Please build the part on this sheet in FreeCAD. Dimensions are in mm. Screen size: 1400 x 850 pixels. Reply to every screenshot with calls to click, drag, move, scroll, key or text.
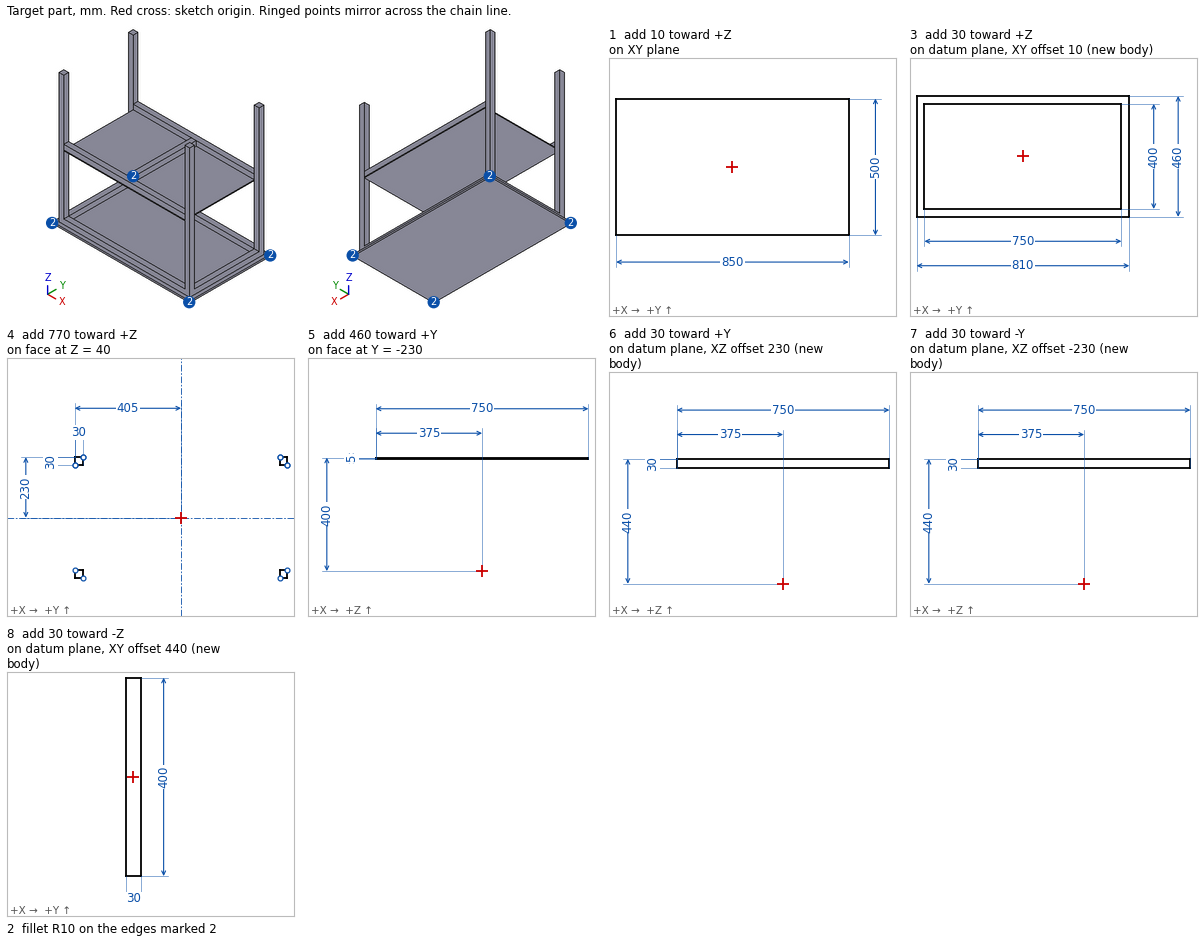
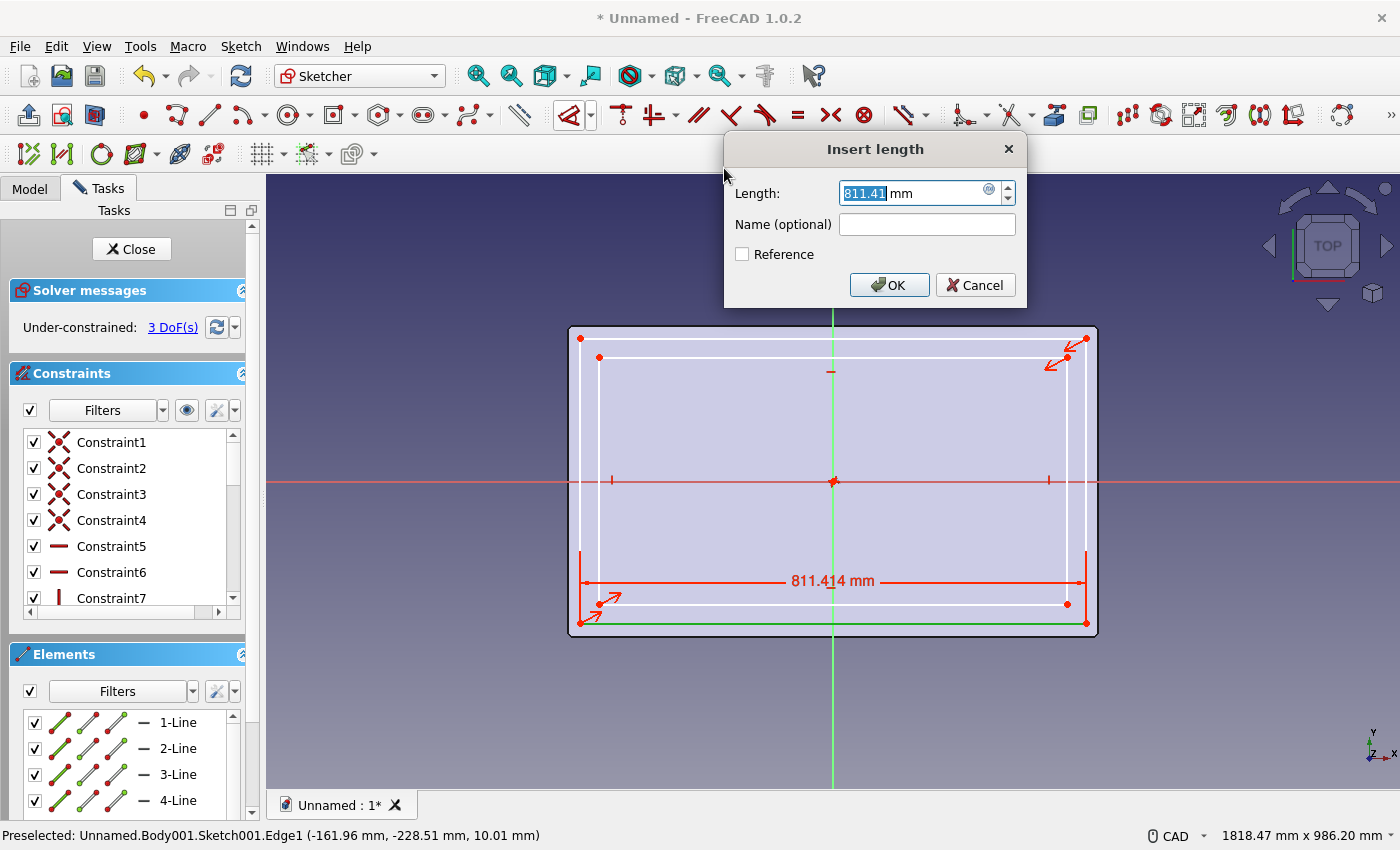
text(810)
key(Return)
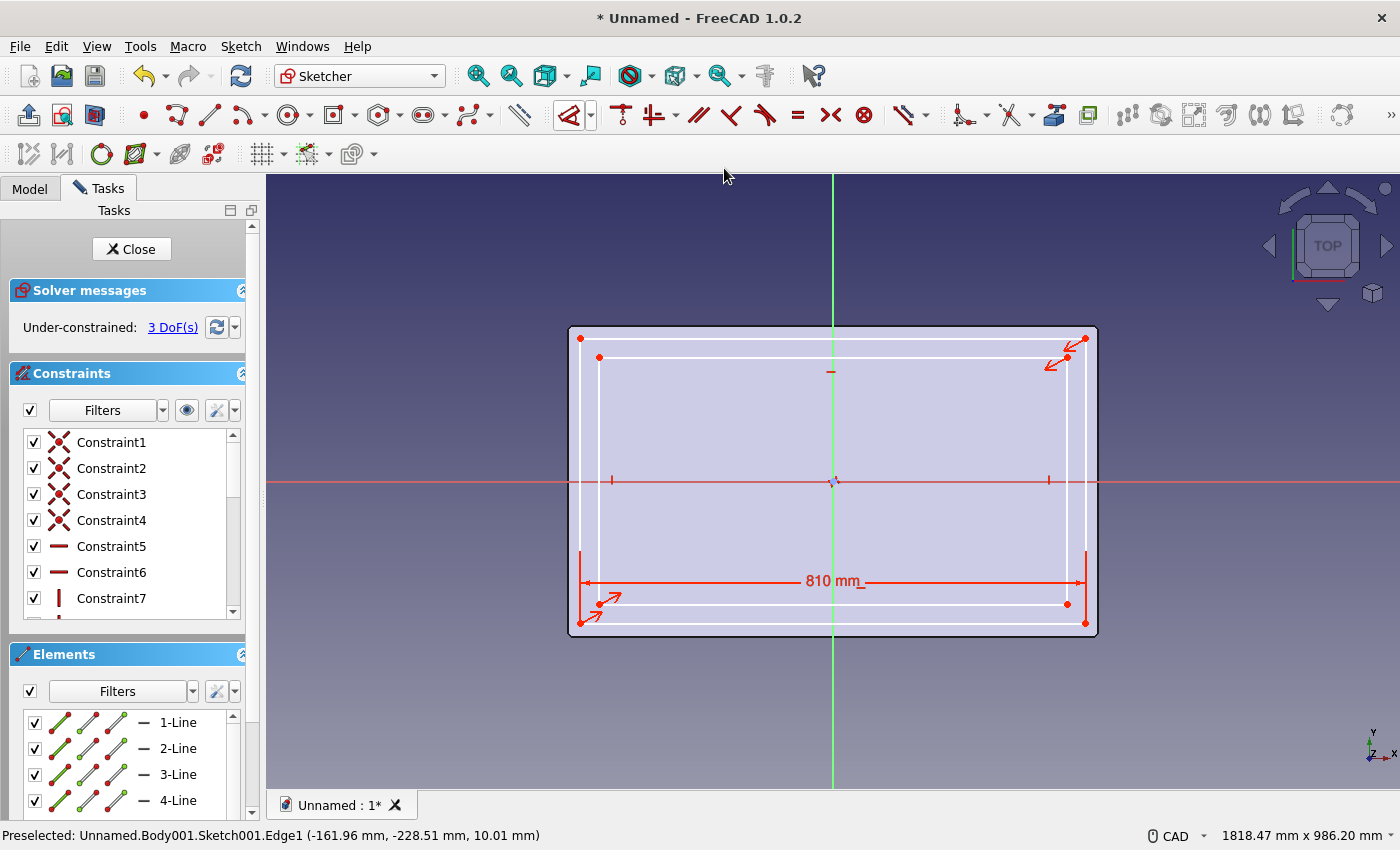
click(1086, 539)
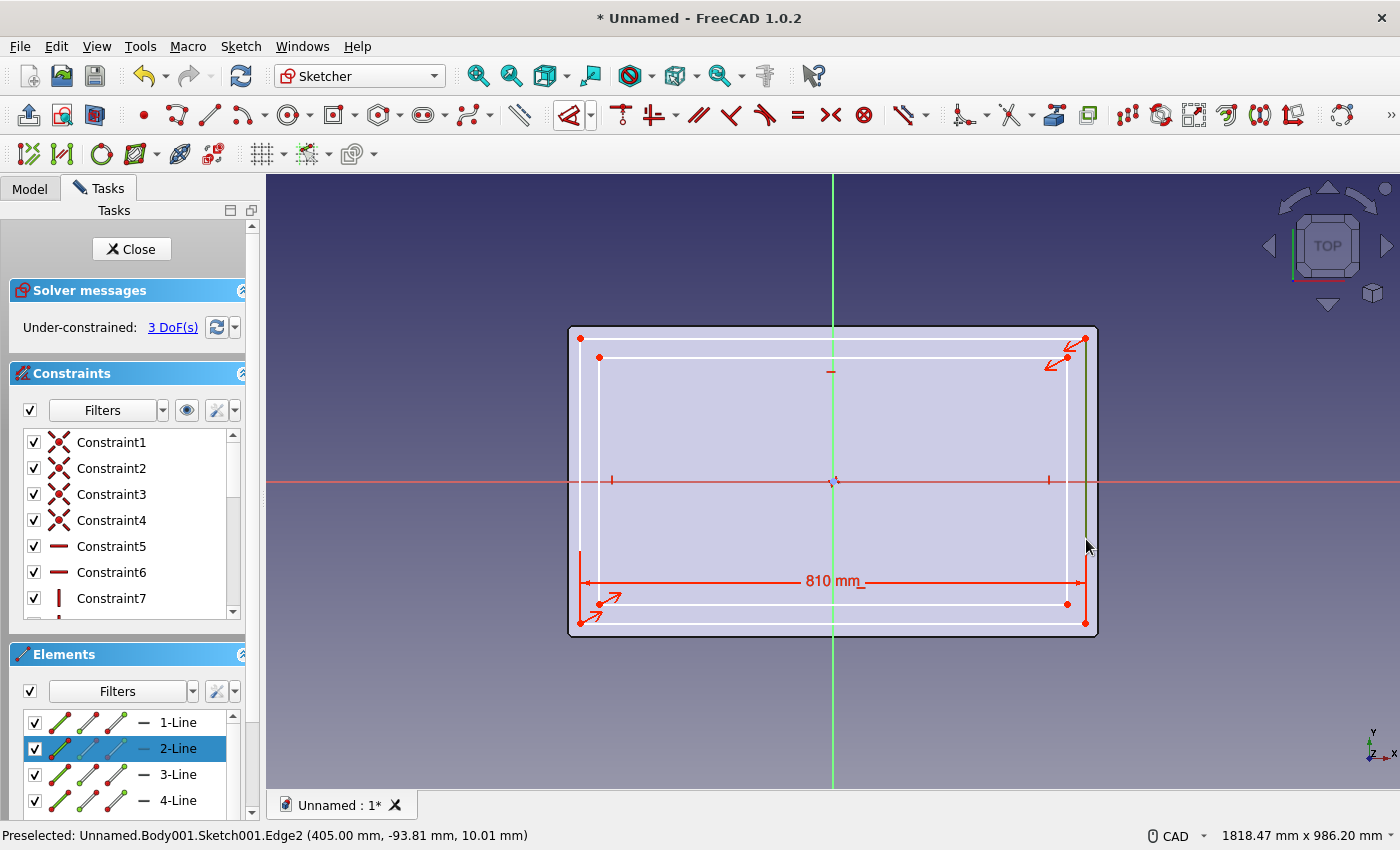
click(590, 116)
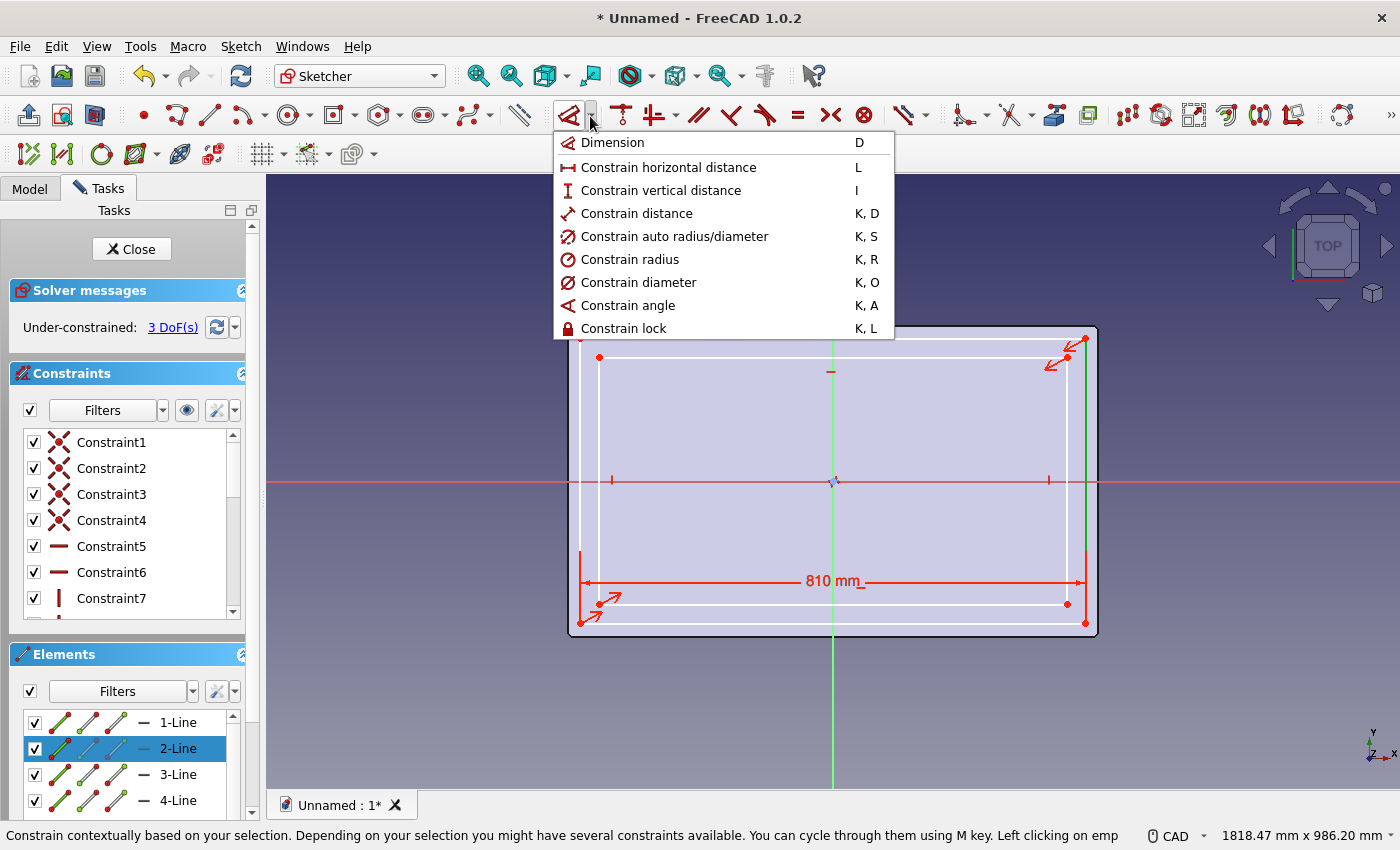
click(724, 190)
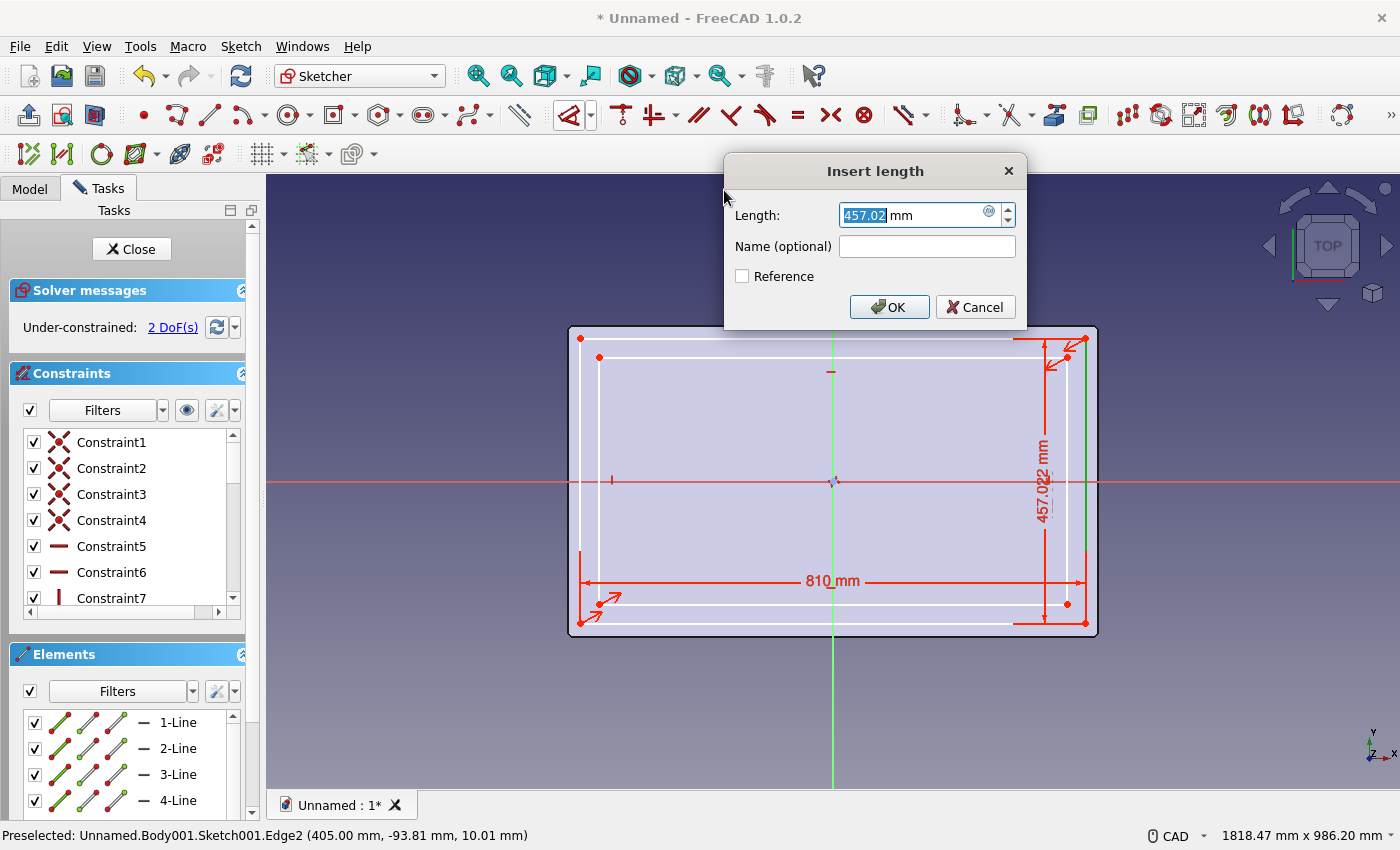
text(460)
key(Return)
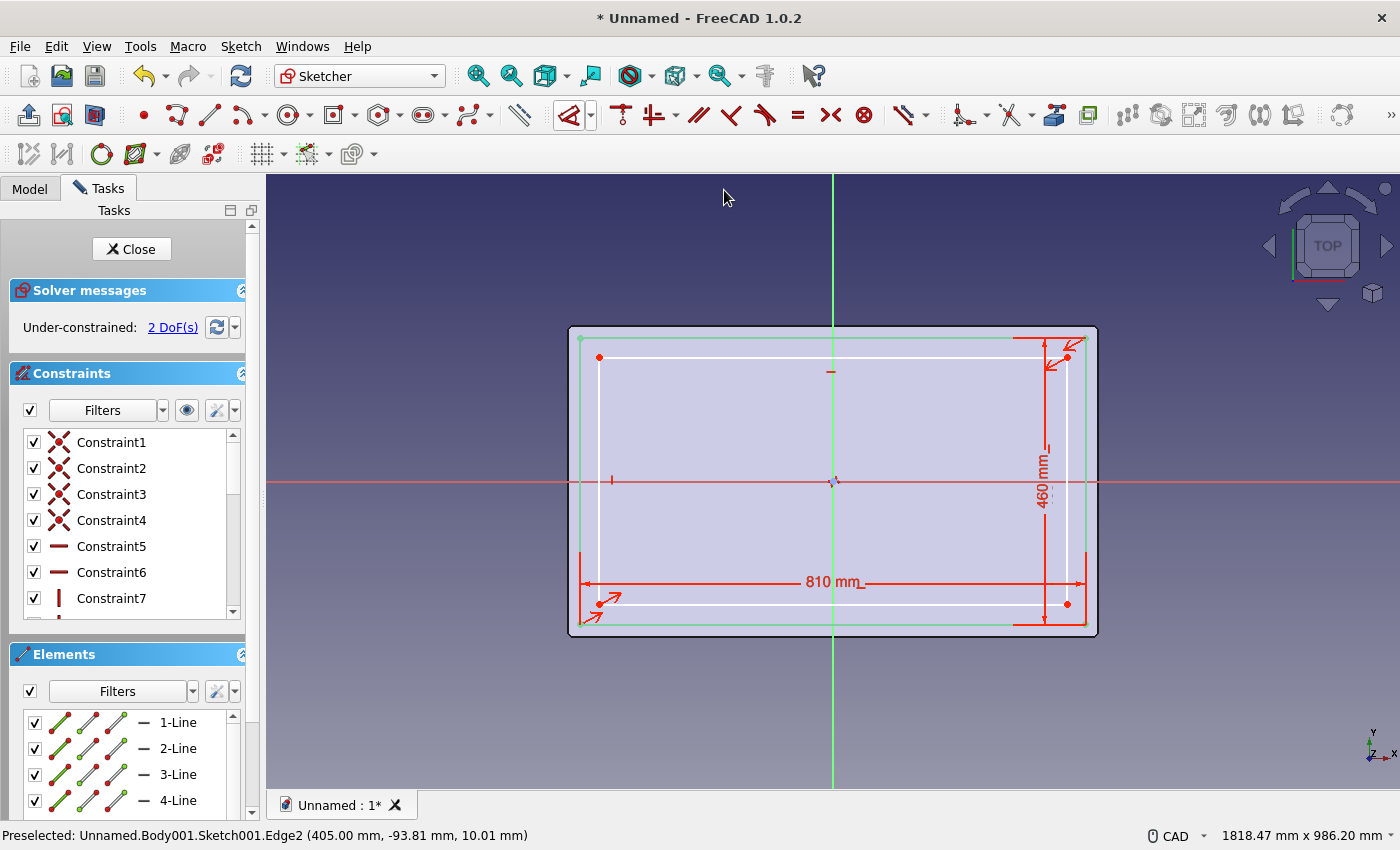
click(739, 605)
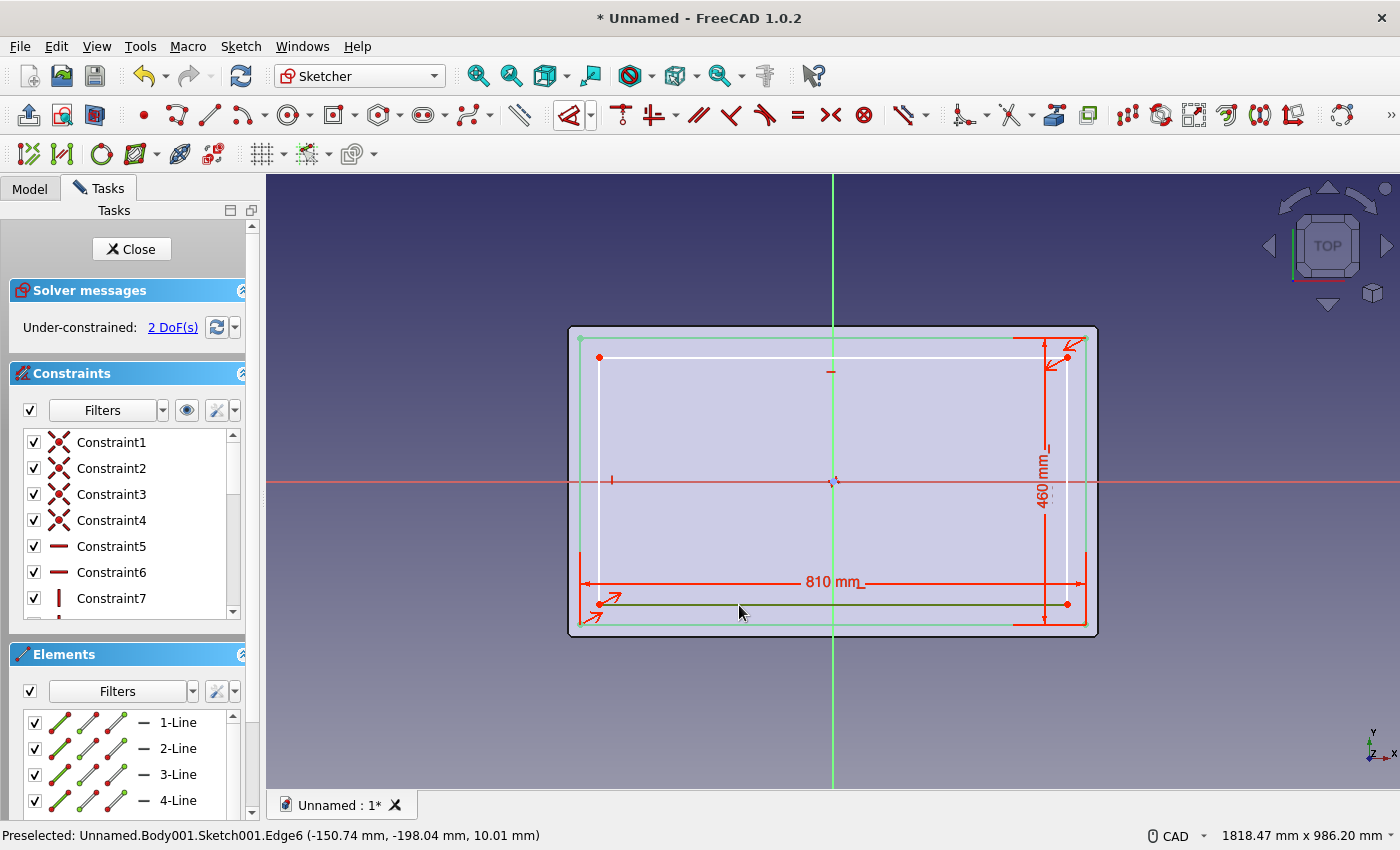
key(l)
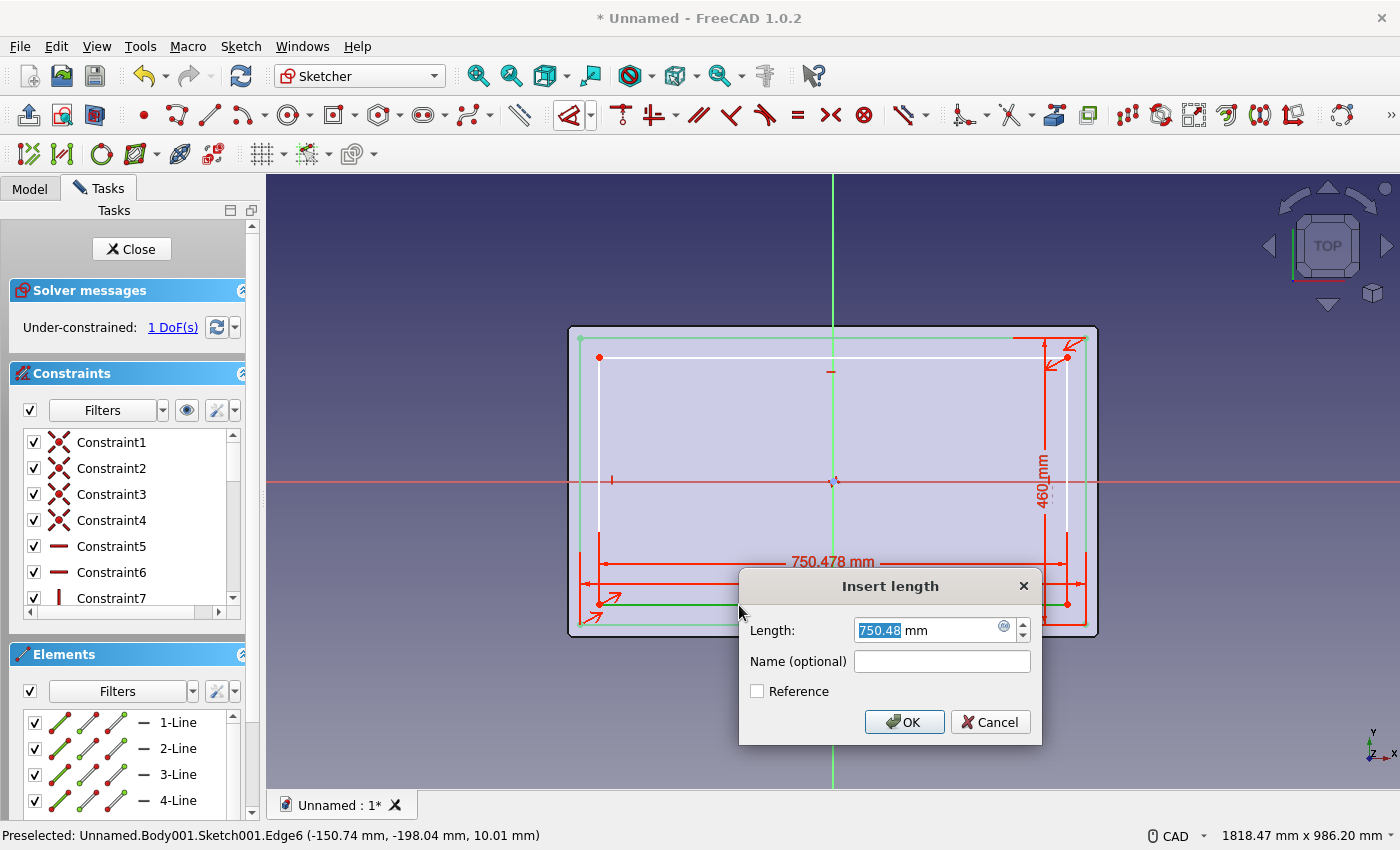
text(750)
key(Return)